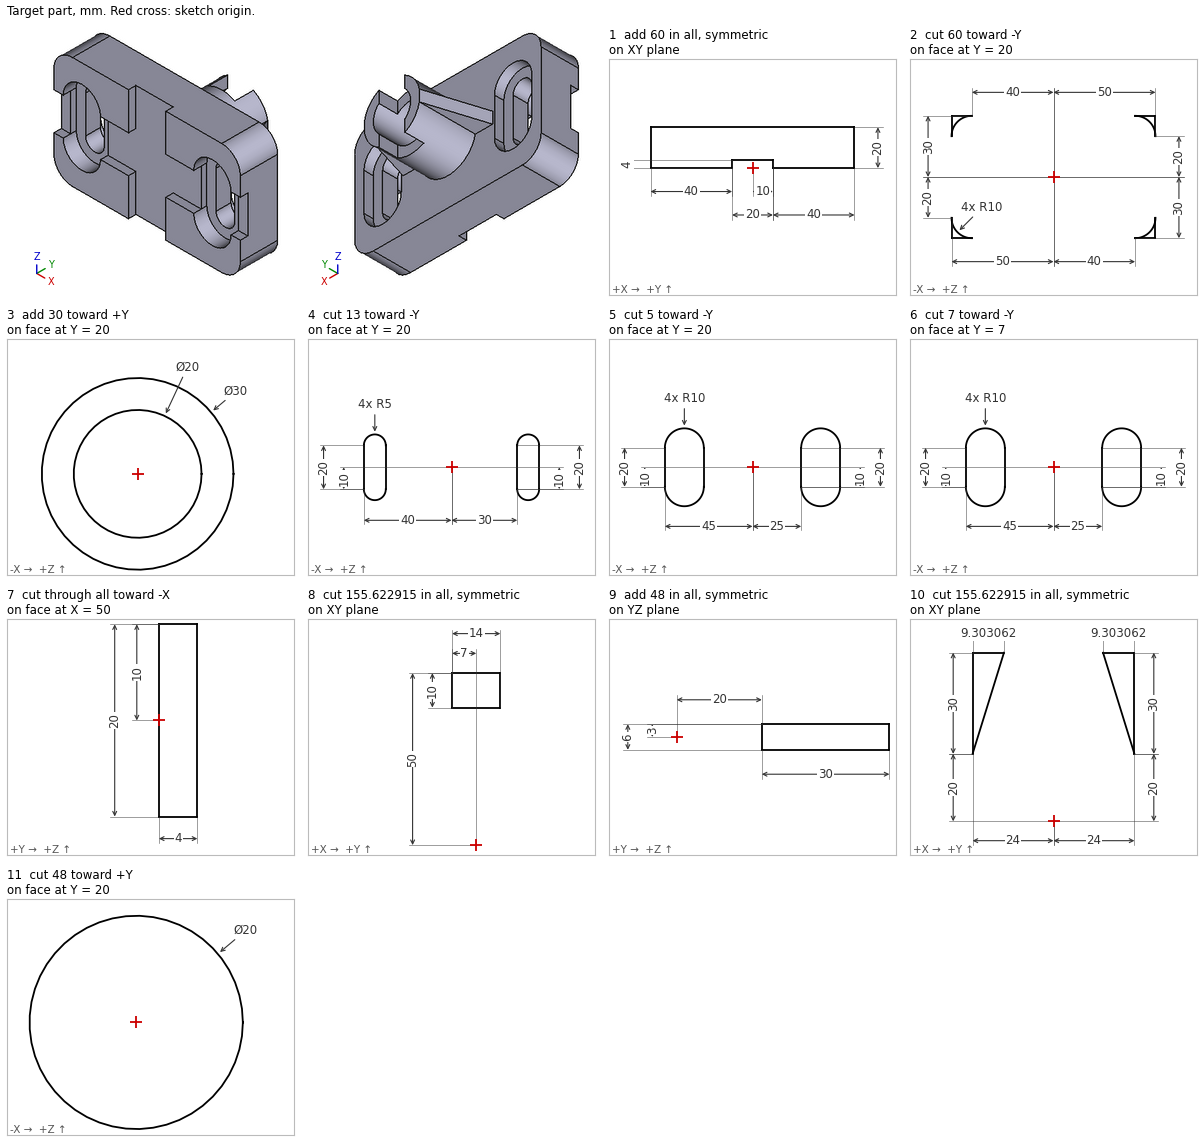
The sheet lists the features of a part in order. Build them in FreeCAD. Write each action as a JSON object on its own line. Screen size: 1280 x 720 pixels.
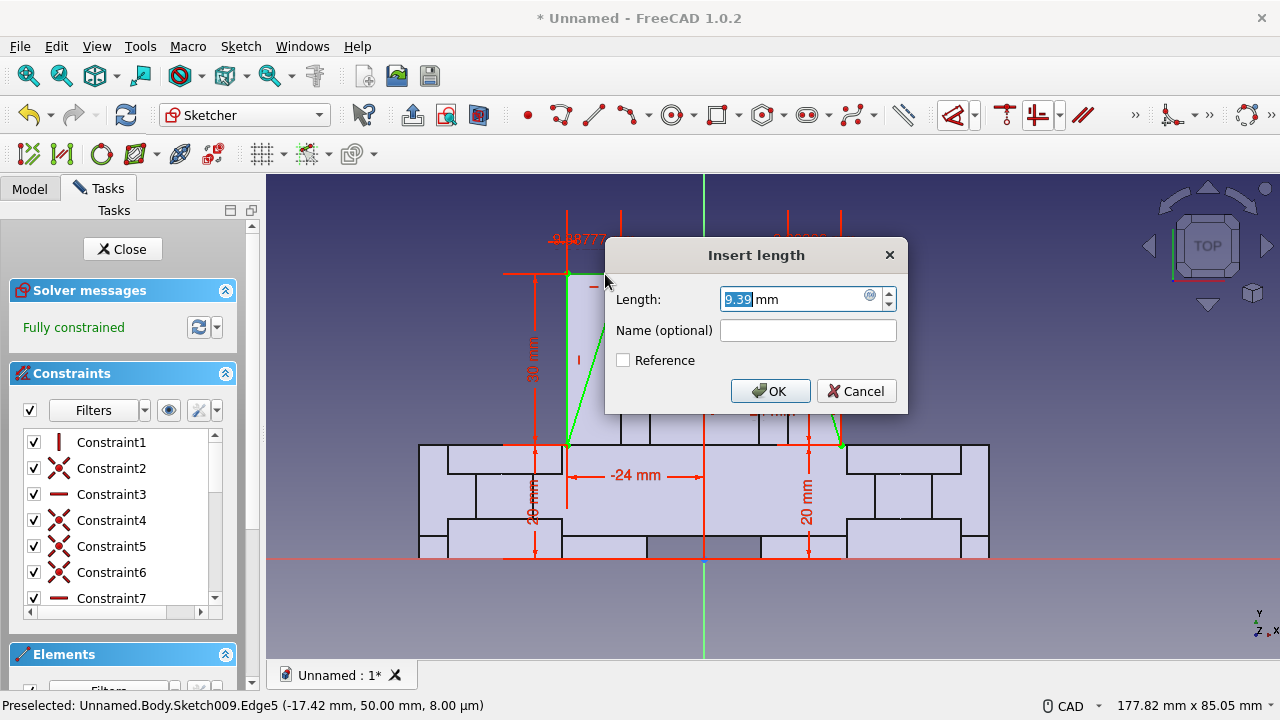
{"action": "type", "text": "9.303062"}
{"action": "key", "text": "Return"}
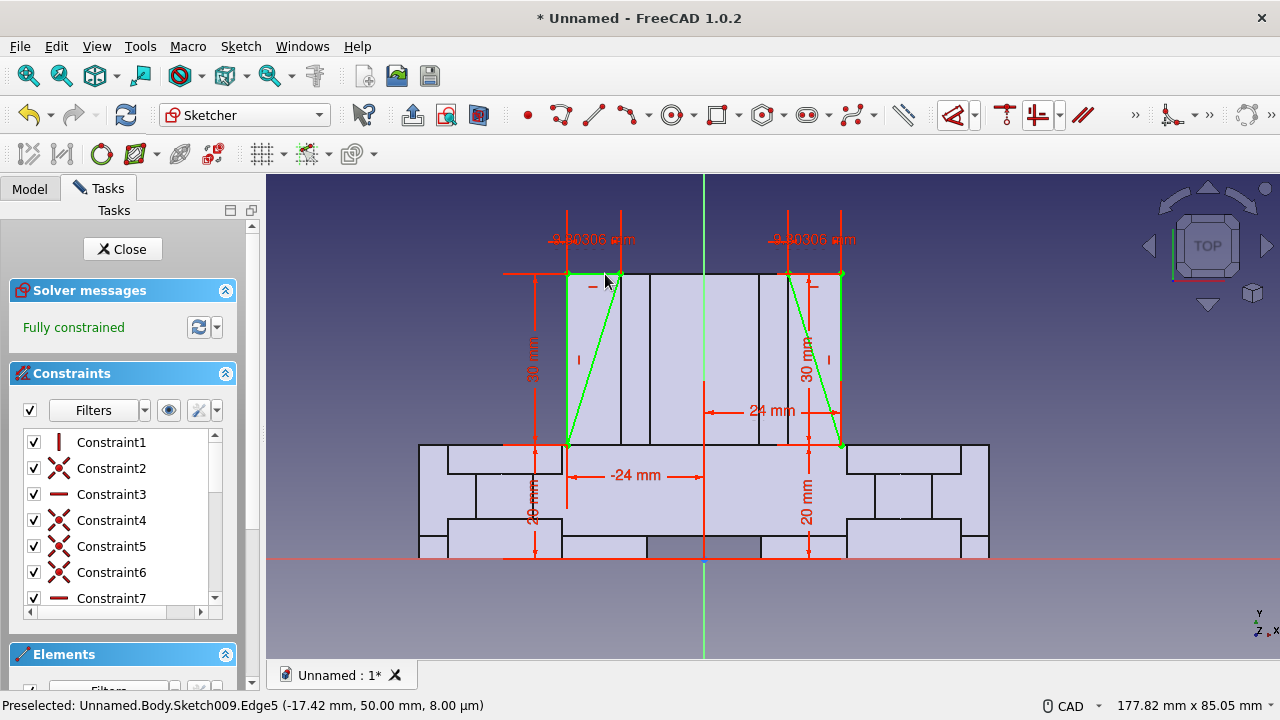
{"action": "left_click", "coordinate": [123, 249]}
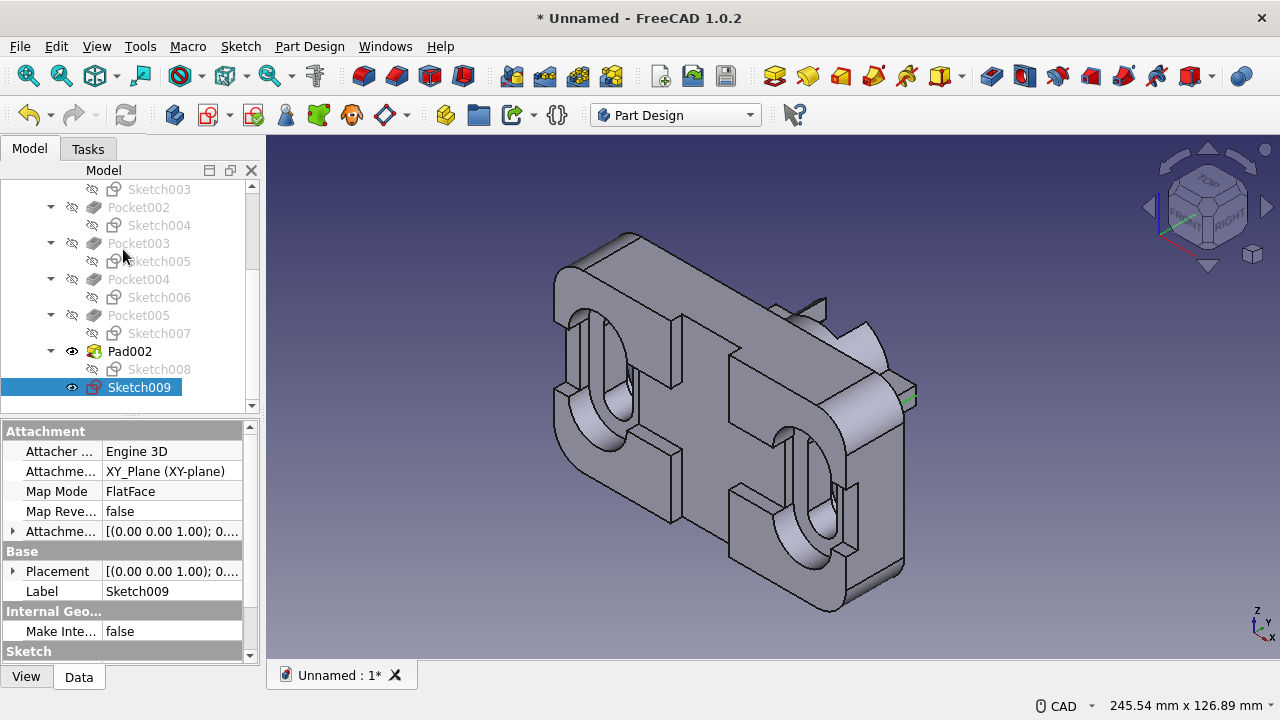
{"action": "left_click", "coordinate": [992, 76]}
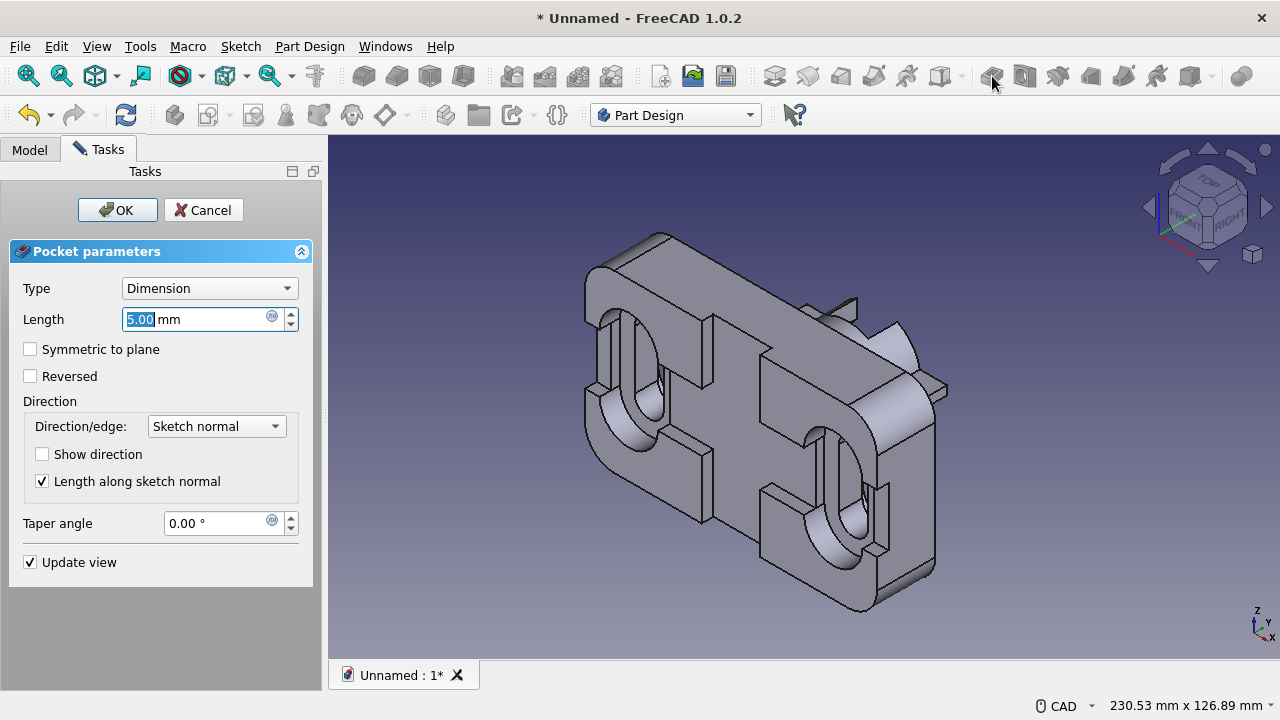
{"action": "type", "text": "155.622915"}
{"action": "key", "text": "Tab"}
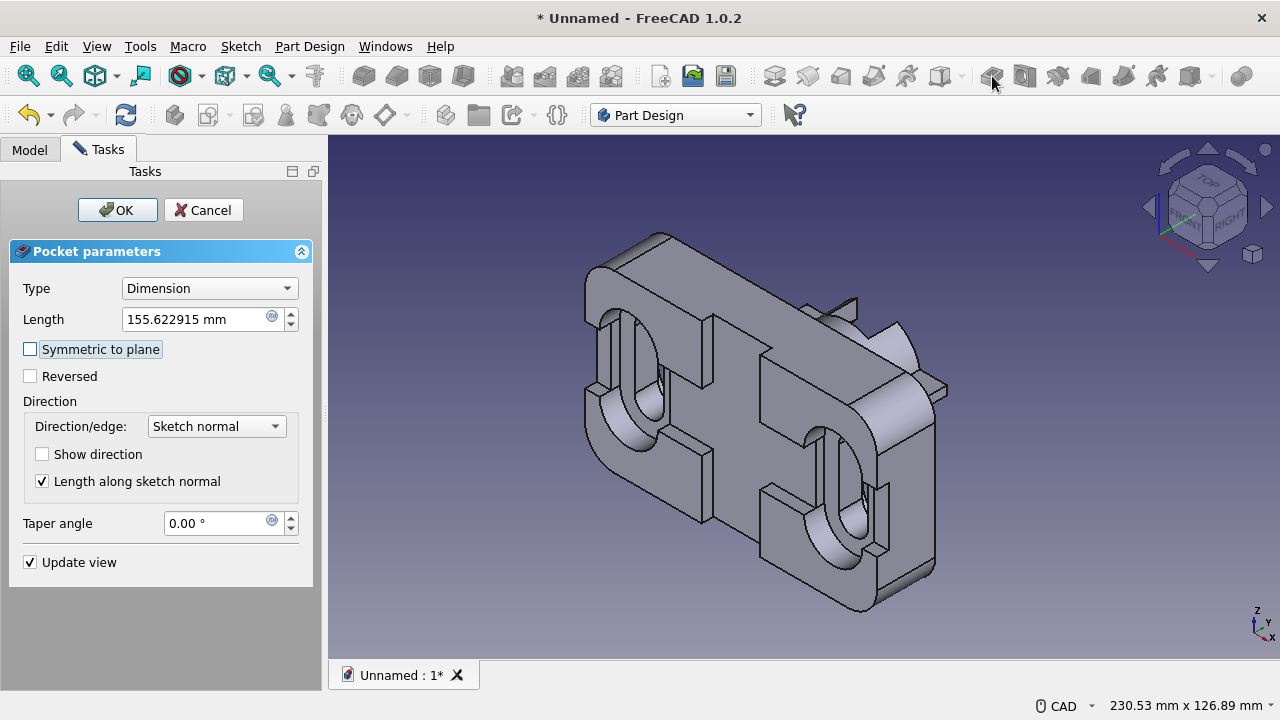
{"action": "left_click", "coordinate": [31, 349]}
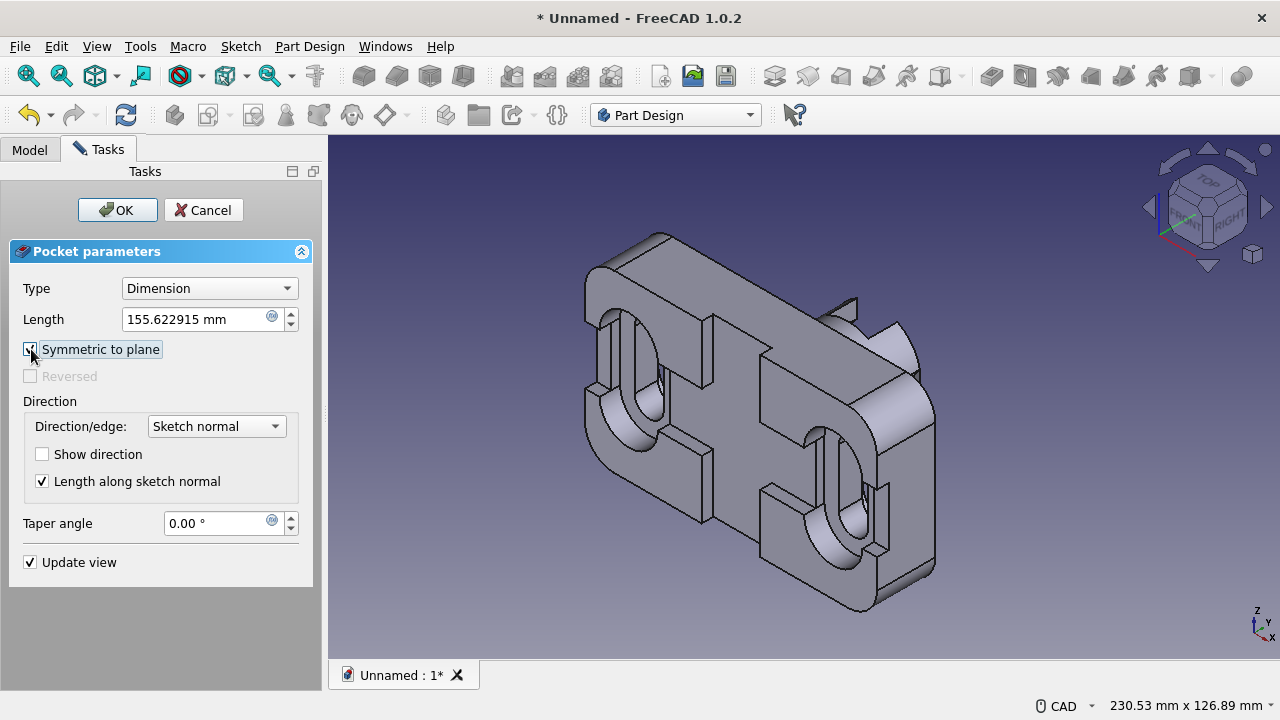
{"action": "left_click", "coordinate": [118, 210]}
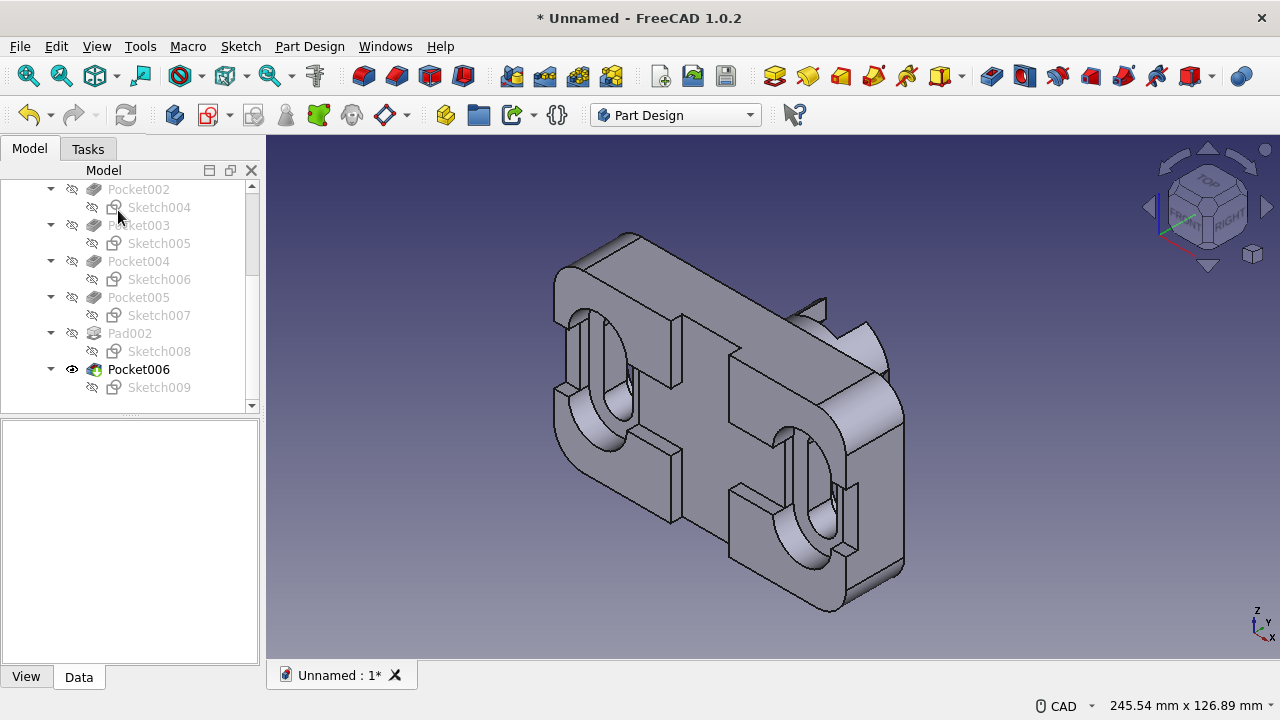
{"action": "key", "text": "4"}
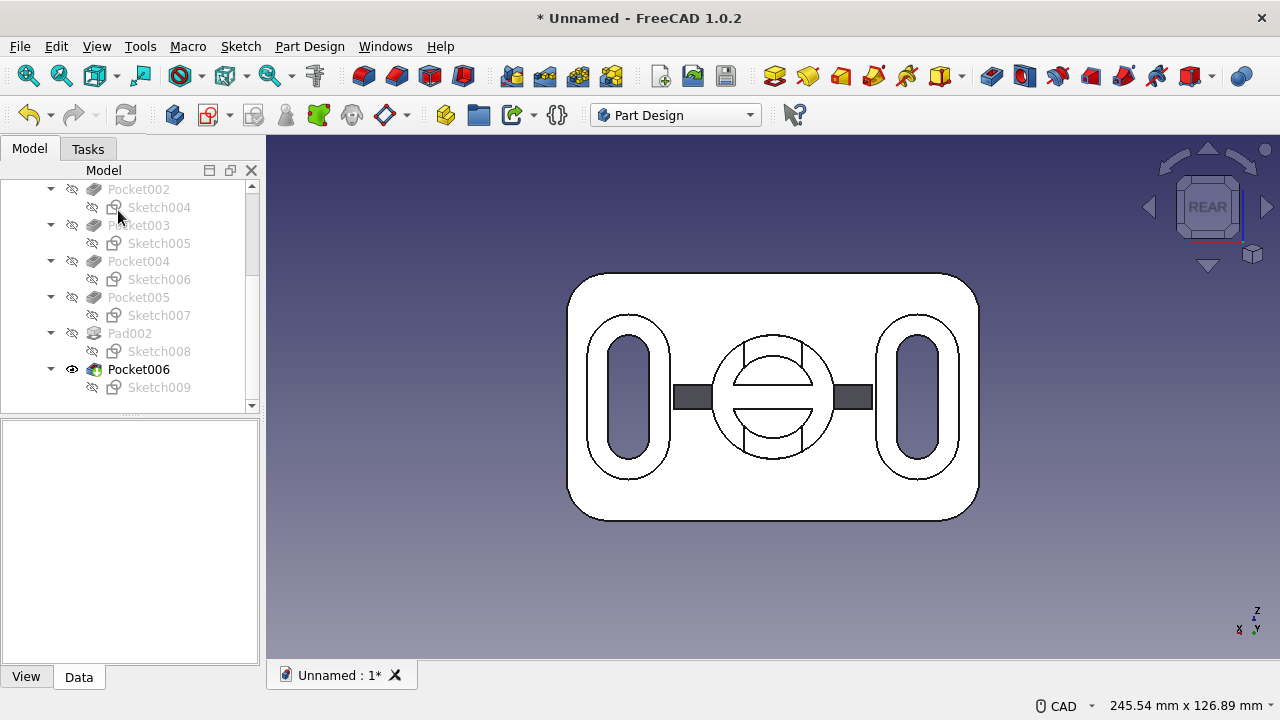
{"action": "left_click", "coordinate": [714, 325]}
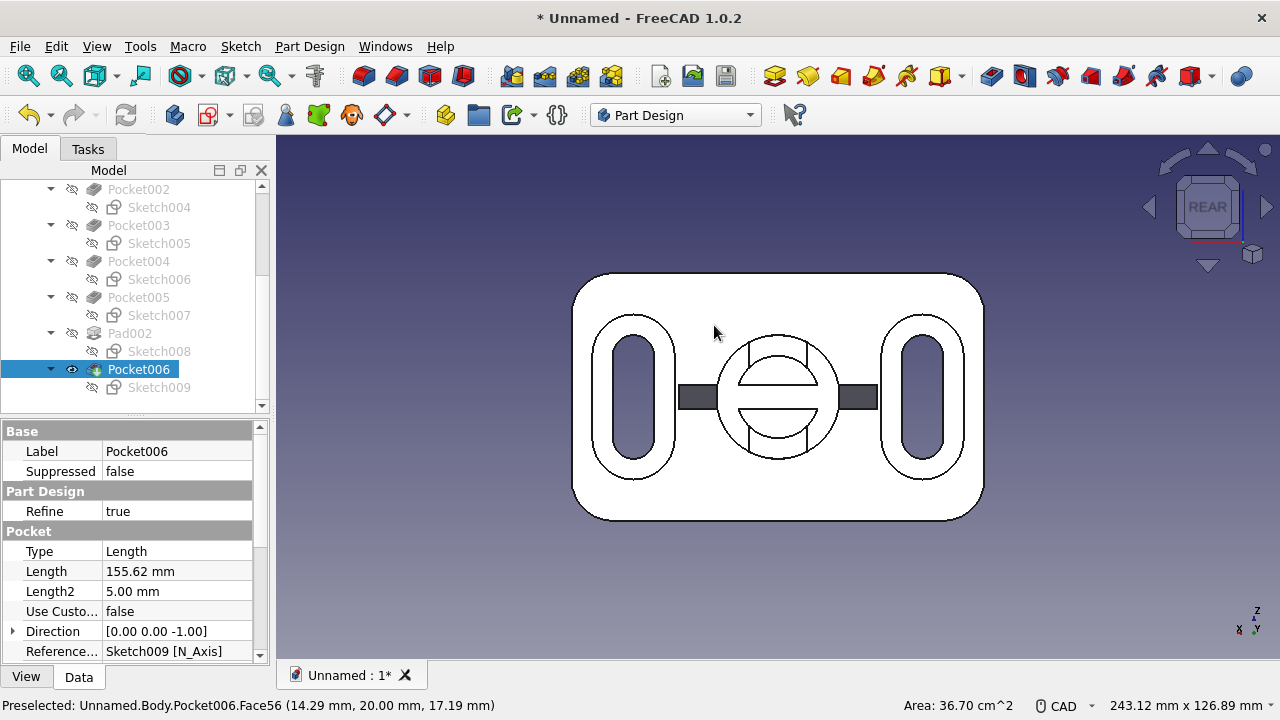
{"action": "left_click", "coordinate": [208, 116]}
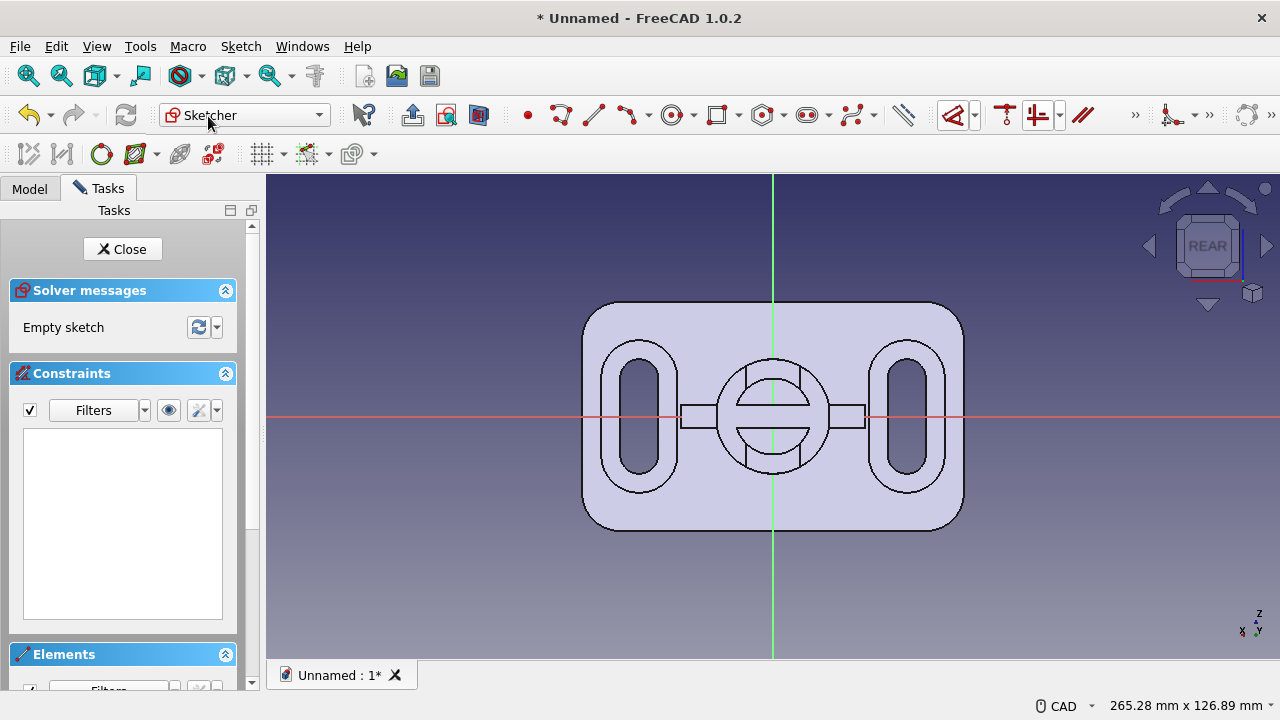
{"action": "key", "text": "q s"}